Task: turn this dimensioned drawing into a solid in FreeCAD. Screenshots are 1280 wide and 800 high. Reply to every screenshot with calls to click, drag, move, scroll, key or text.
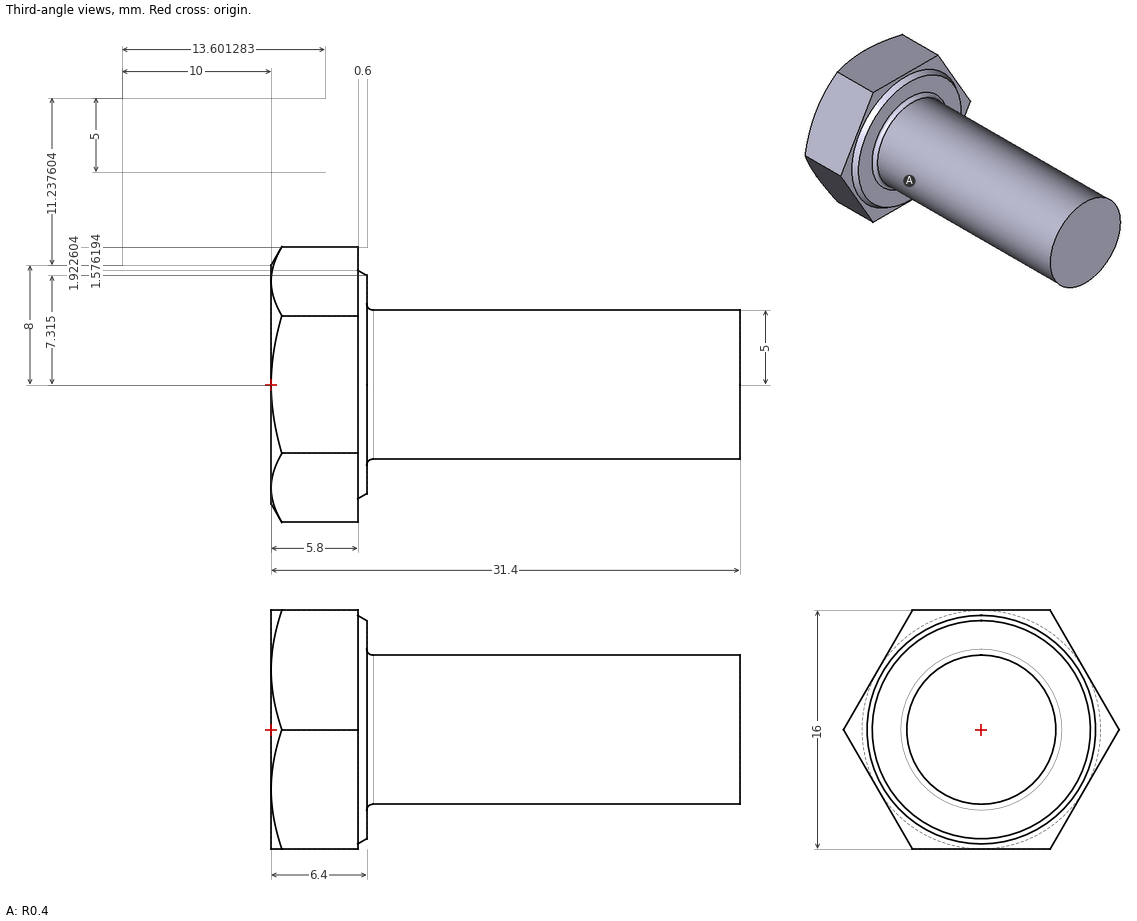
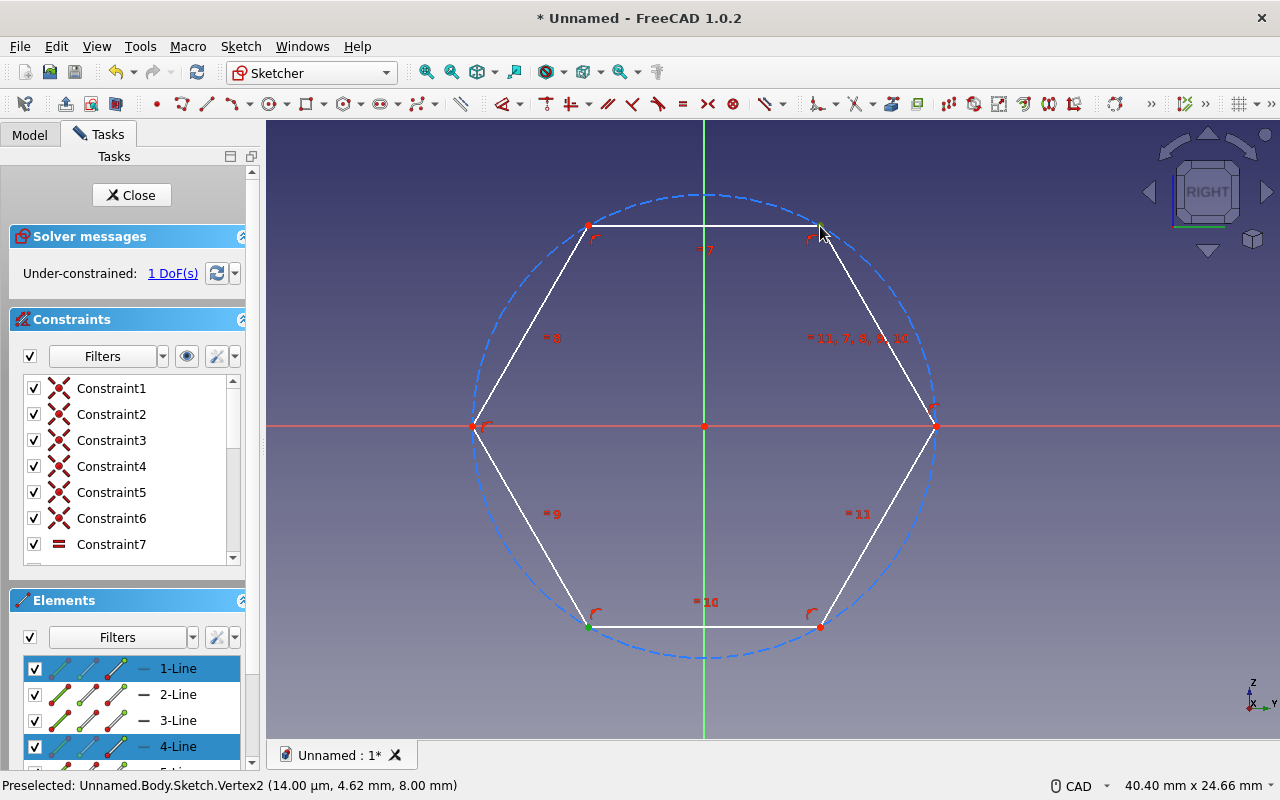
click(520, 104)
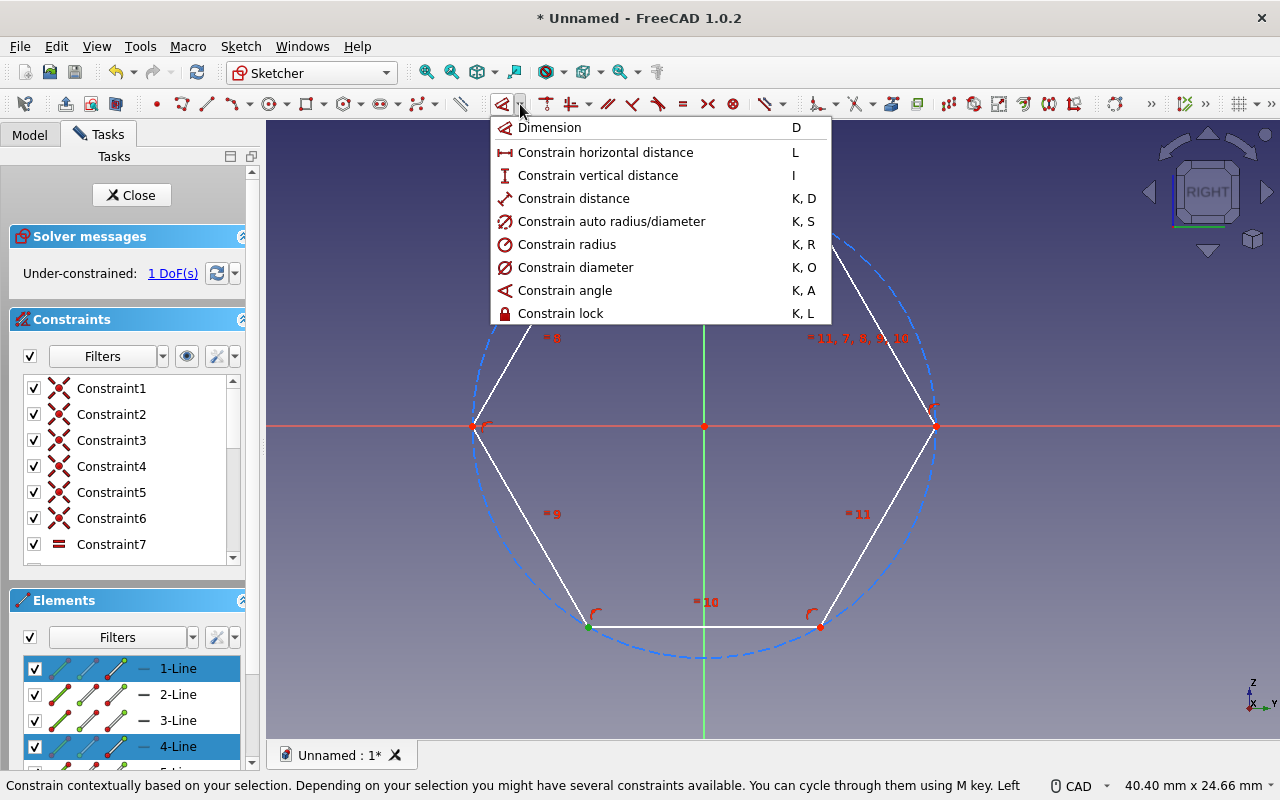
click(661, 176)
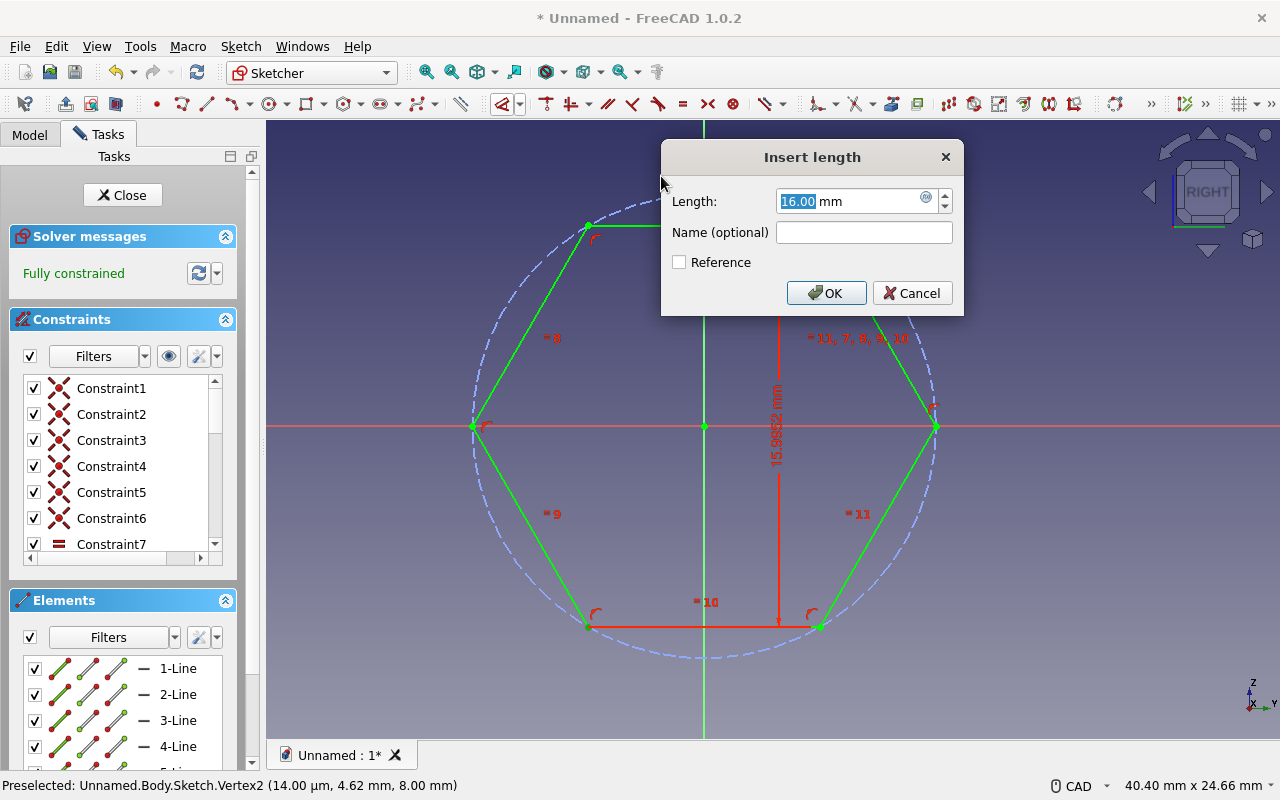
text(16)
key(Return)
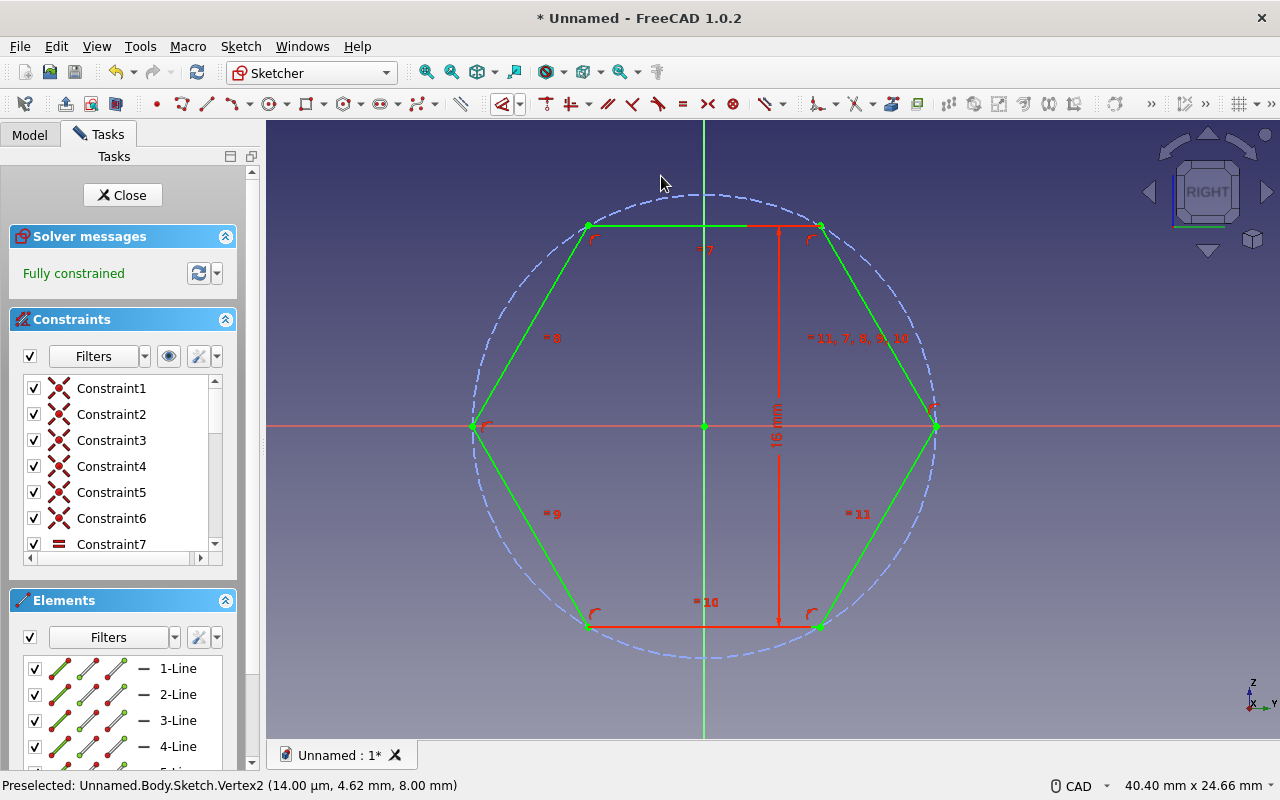
click(123, 195)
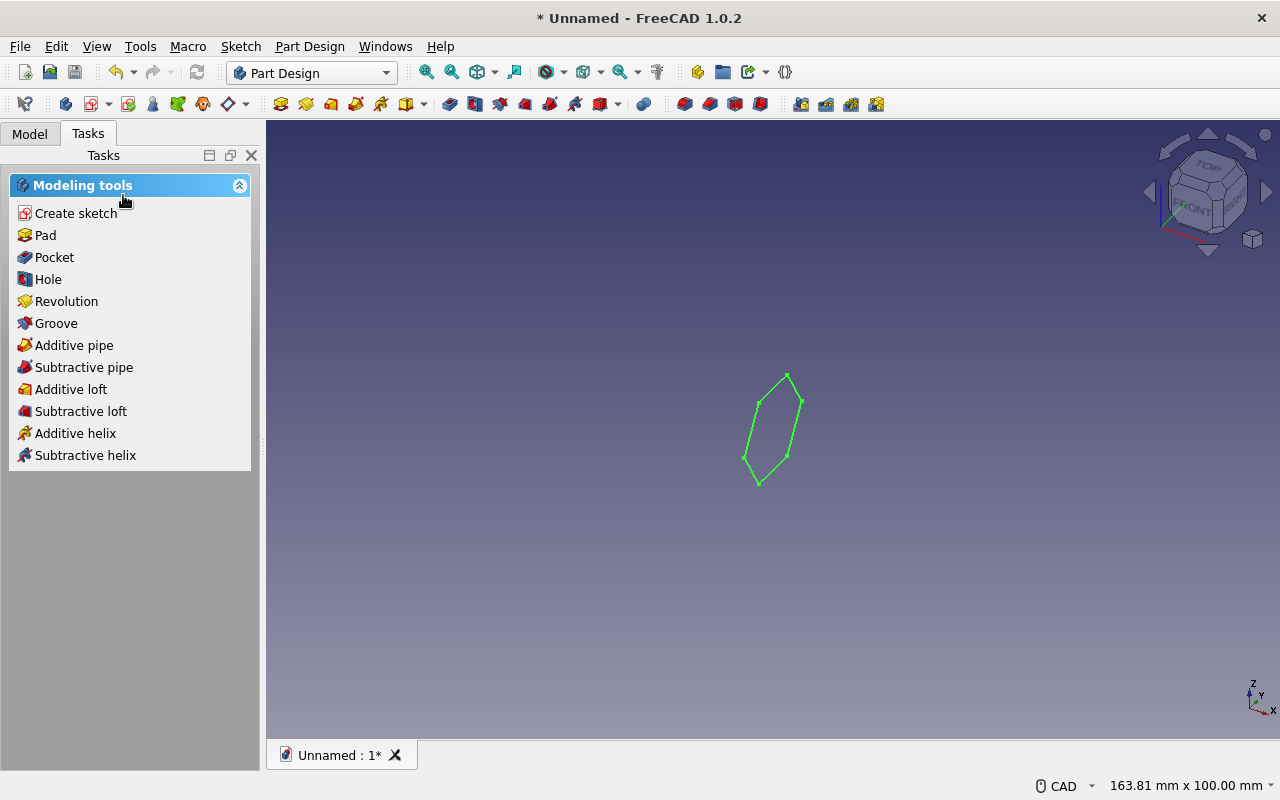
click(281, 104)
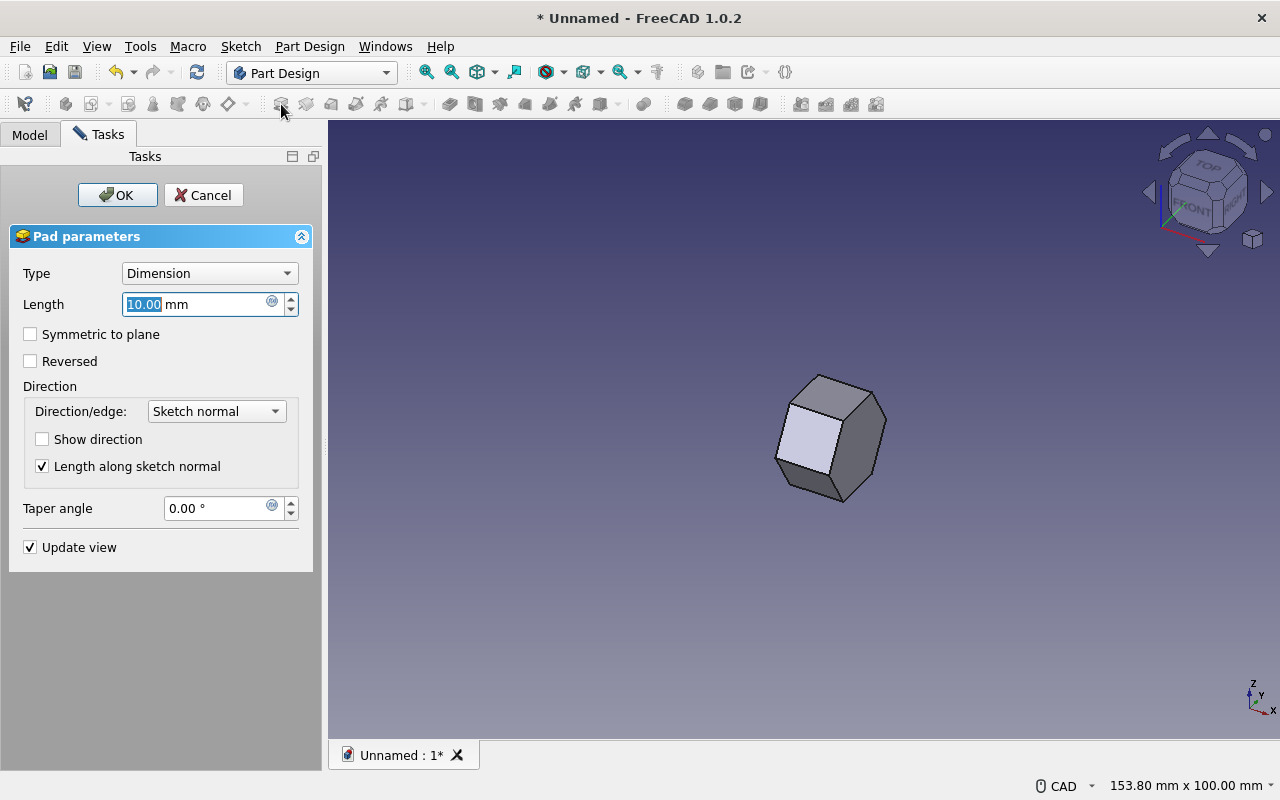
text(6.4)
key(Tab)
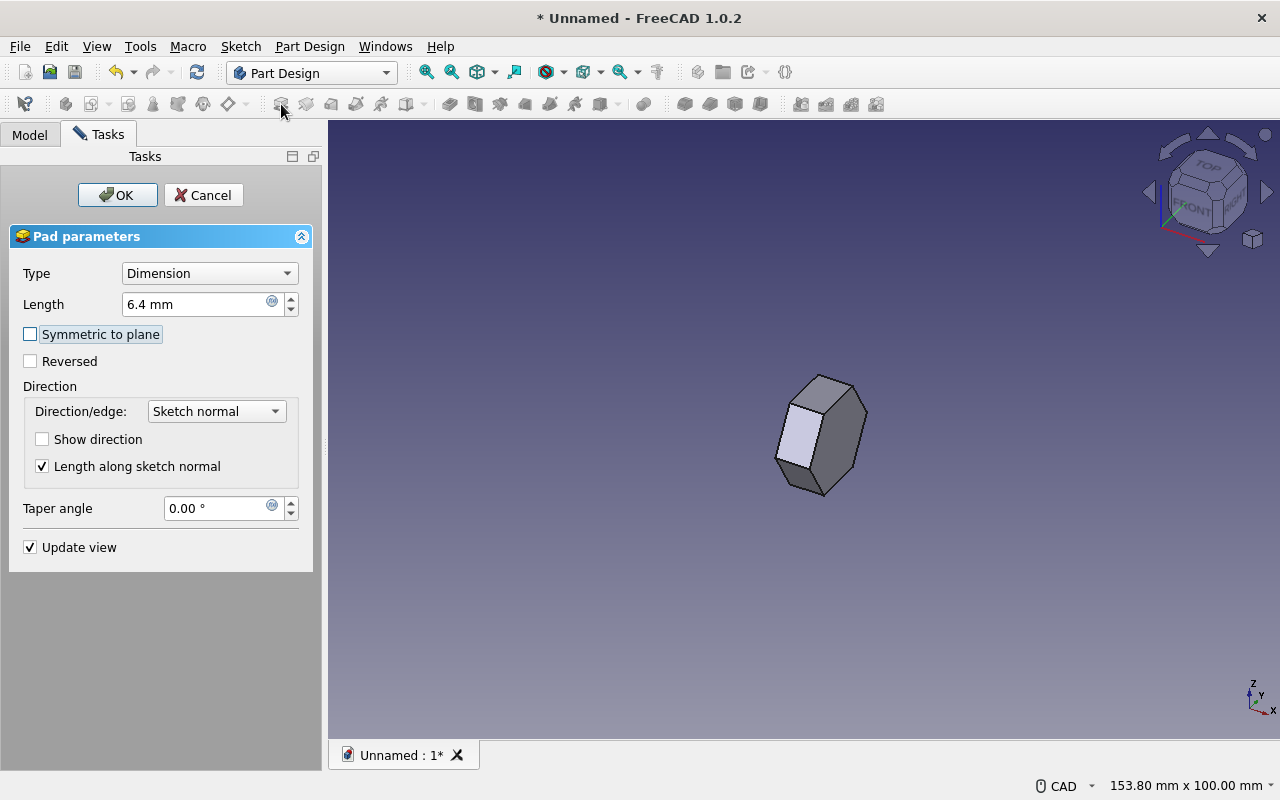
click(118, 195)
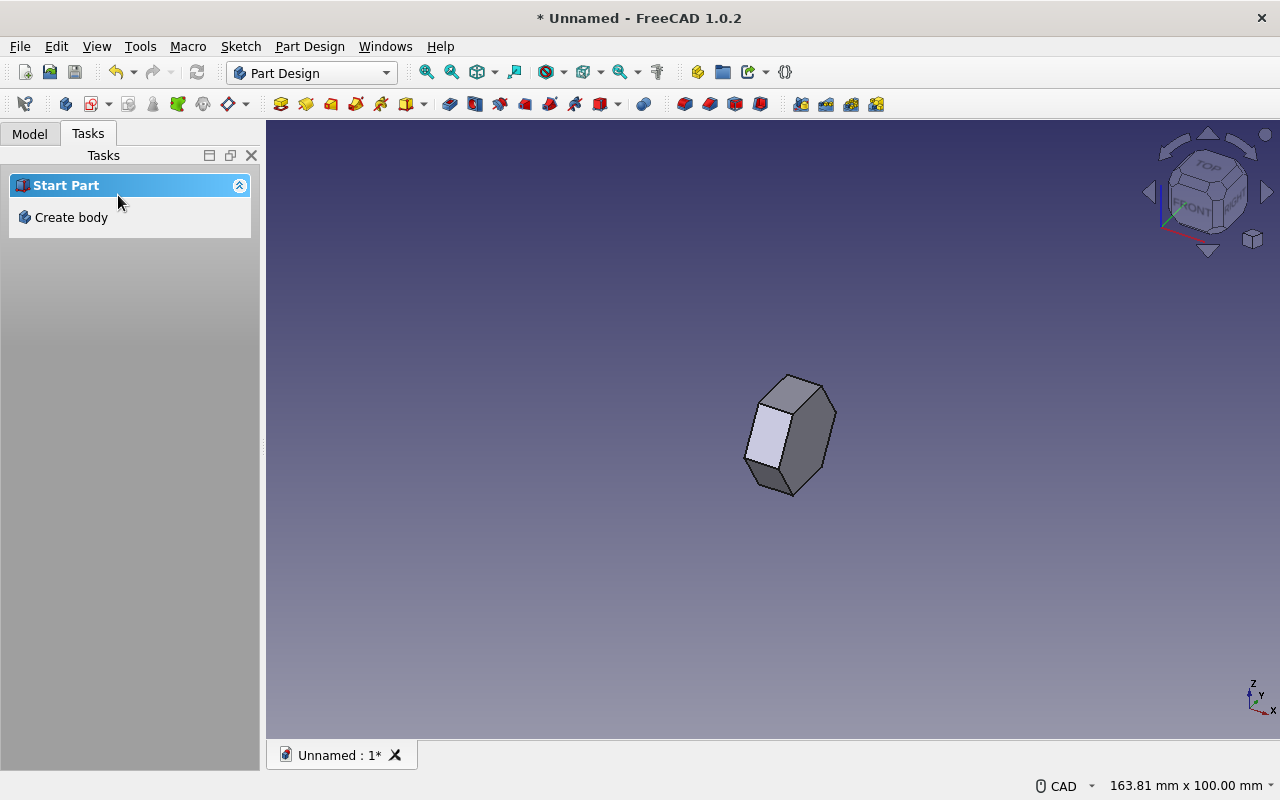
click(427, 72)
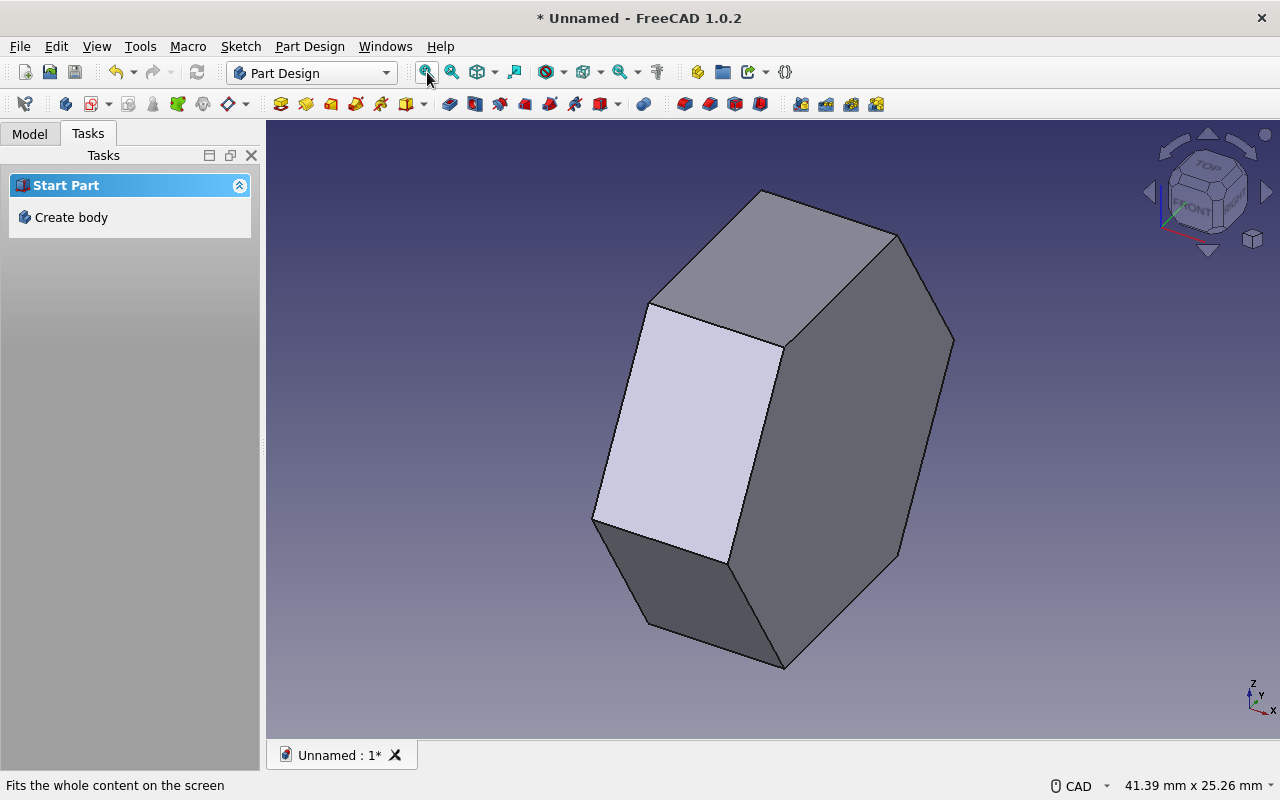
click(90, 104)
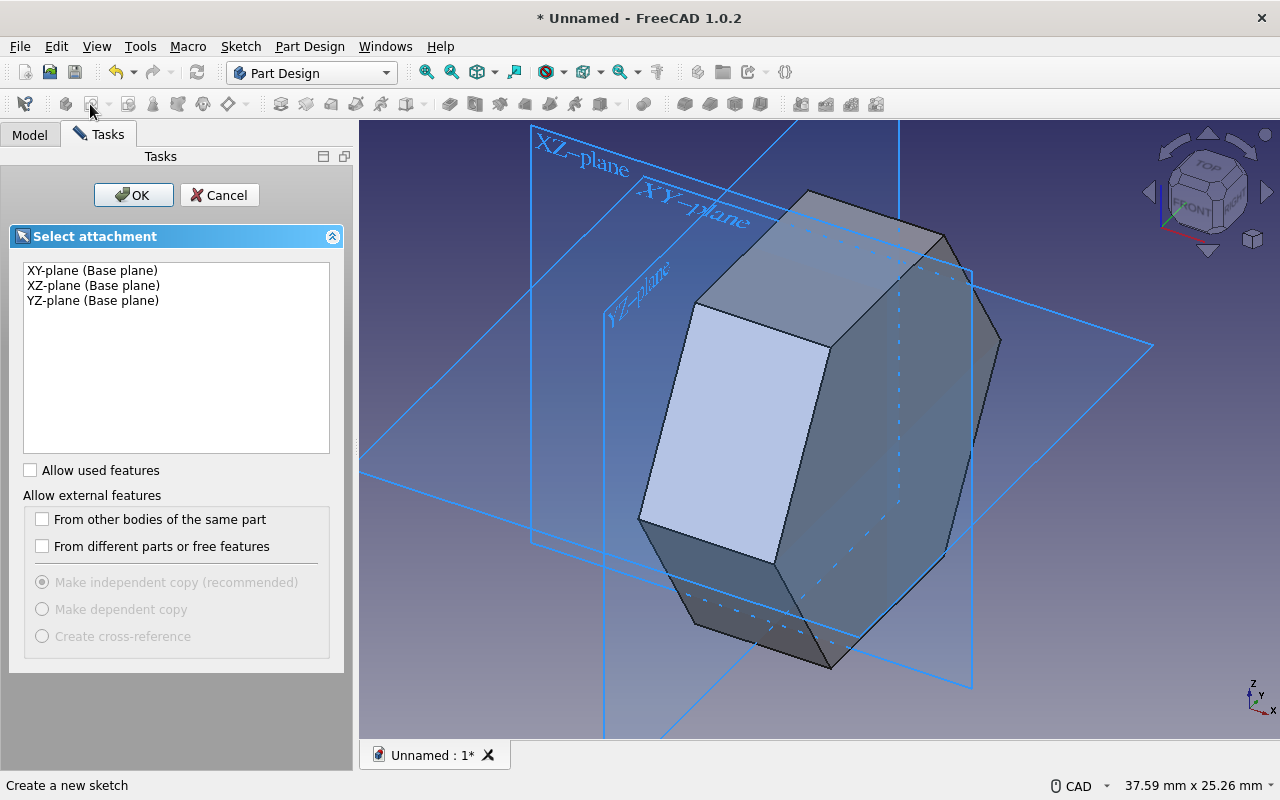
click(84, 270)